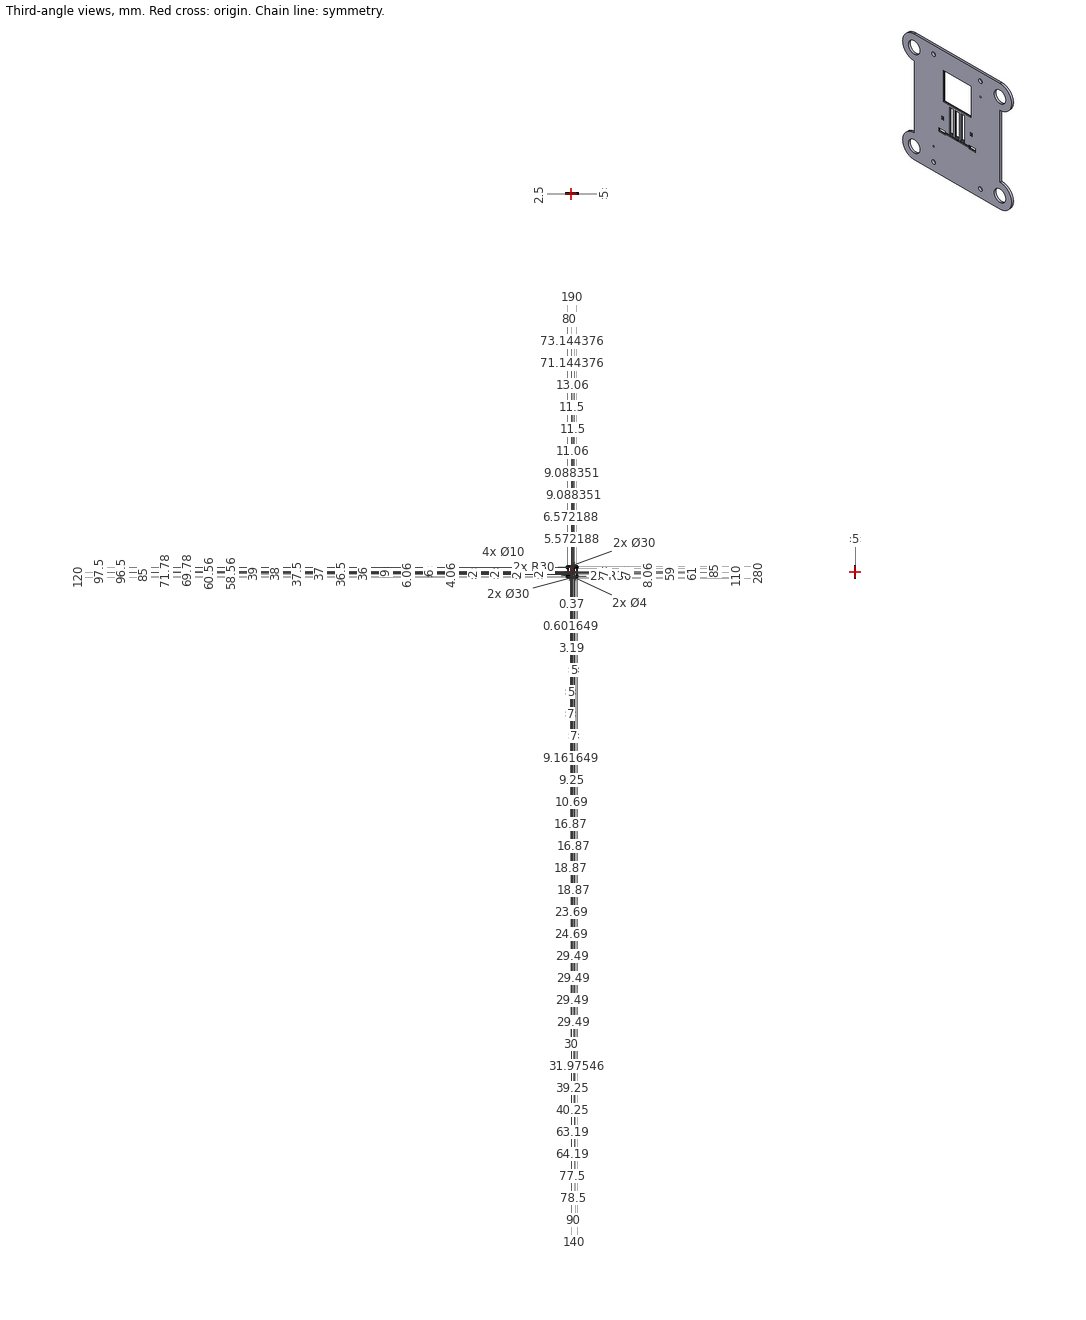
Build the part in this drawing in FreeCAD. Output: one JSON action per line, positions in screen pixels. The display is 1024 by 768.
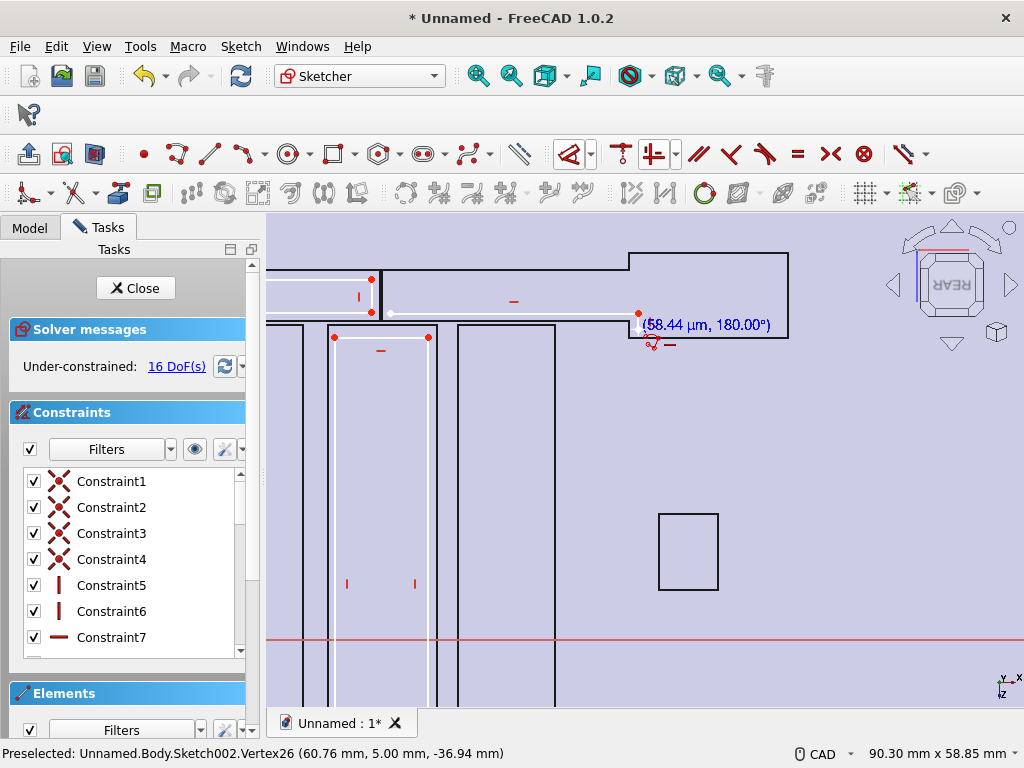
{"action": "scroll", "coordinate": [641, 330], "scroll_direction": "down", "scroll_amount": 7}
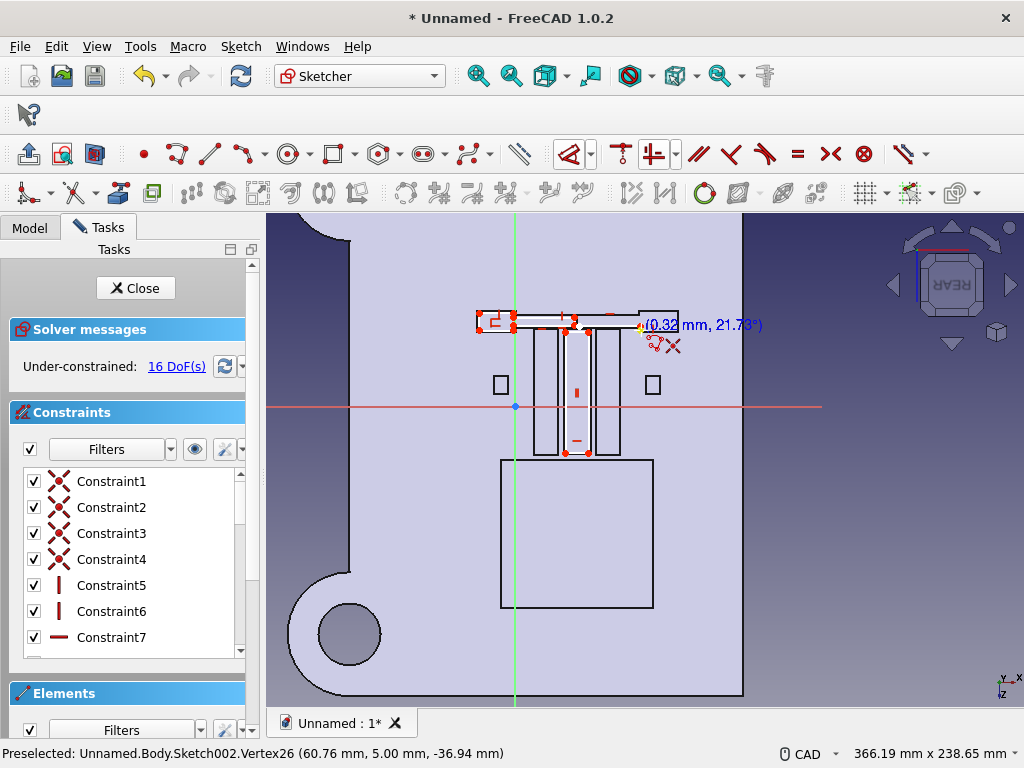
{"action": "left_click", "coordinate": [676, 330]}
{"action": "left_click", "coordinate": [676, 313]}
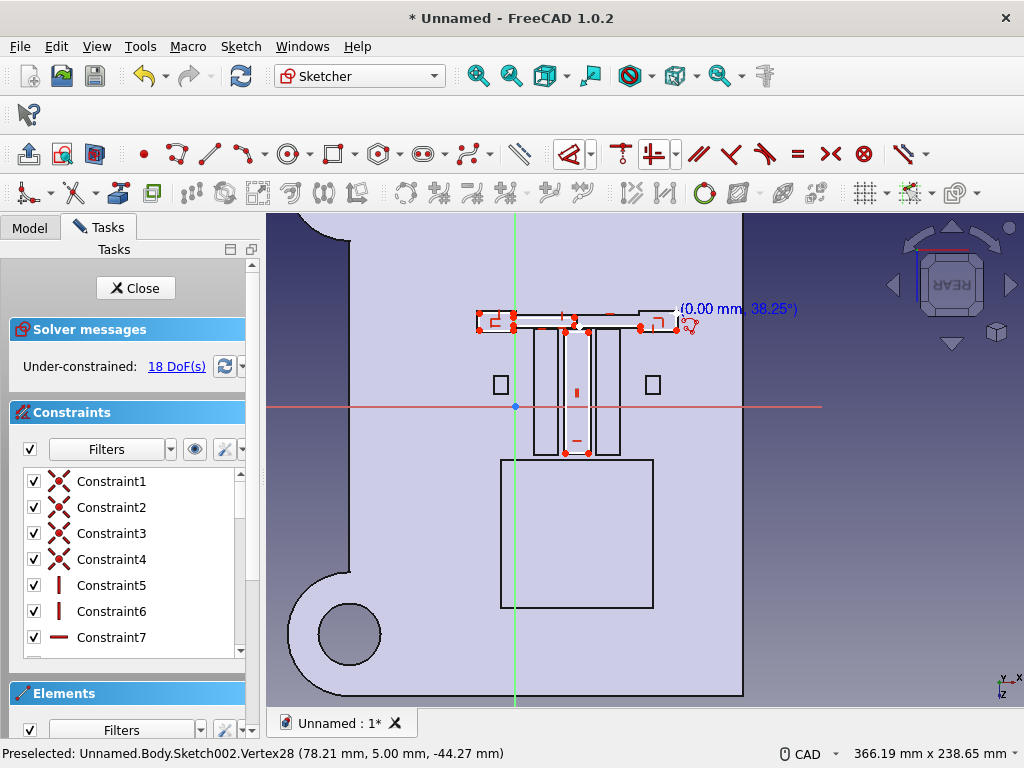
{"action": "scroll", "coordinate": [641, 313], "scroll_direction": "up", "scroll_amount": 2}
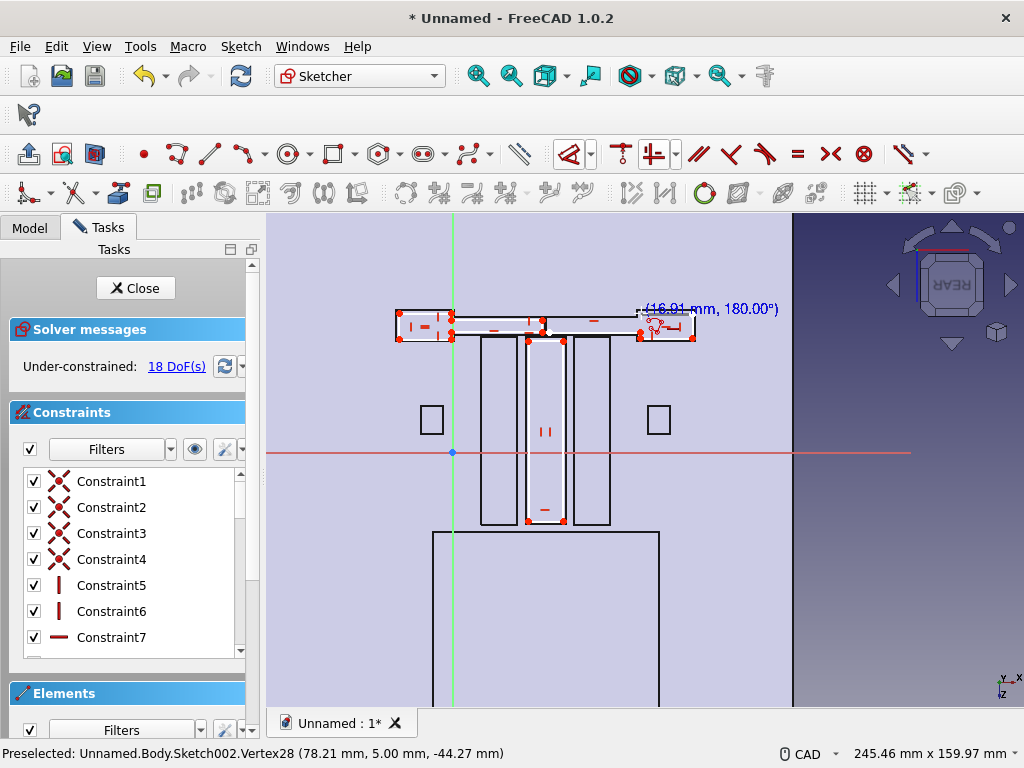
{"action": "left_click", "coordinate": [640, 313]}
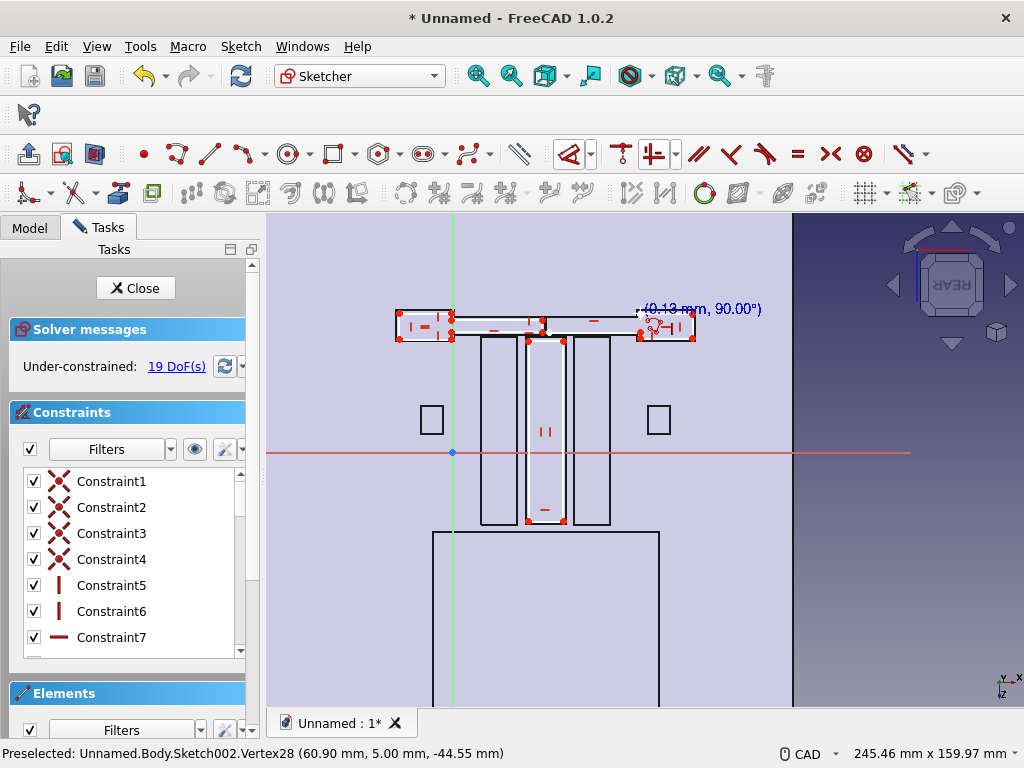
{"action": "scroll", "coordinate": [640, 320], "scroll_direction": "up", "scroll_amount": 5}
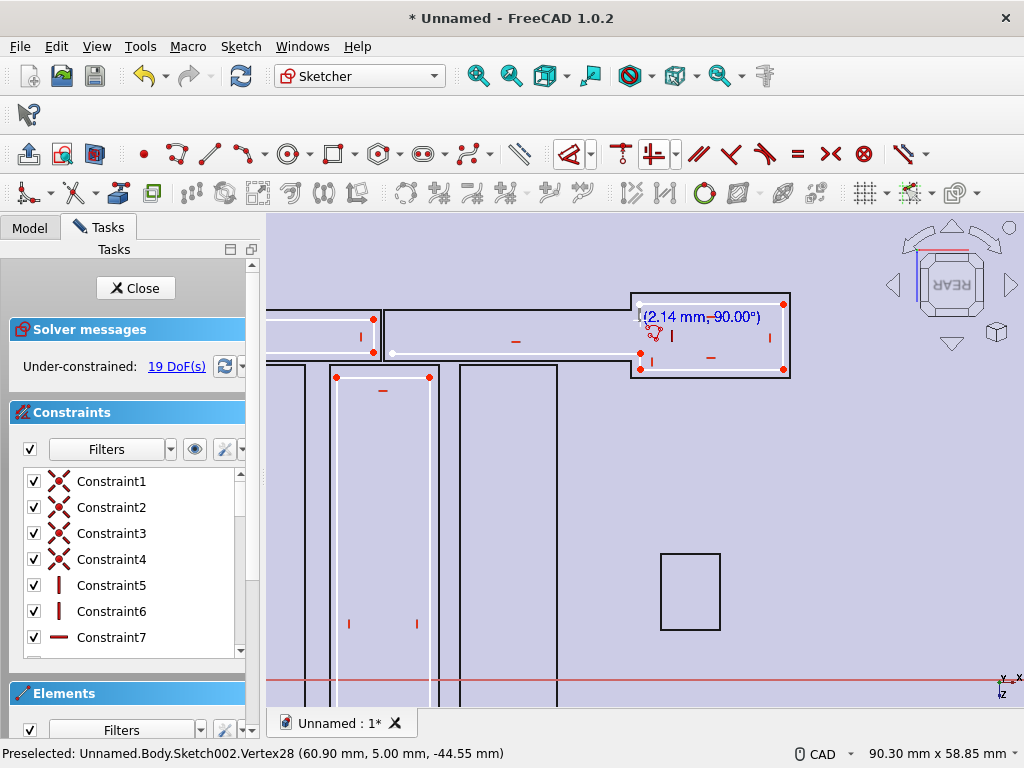
{"action": "left_click", "coordinate": [639, 319]}
{"action": "left_click", "coordinate": [392, 319]}
{"action": "left_click", "coordinate": [392, 354]}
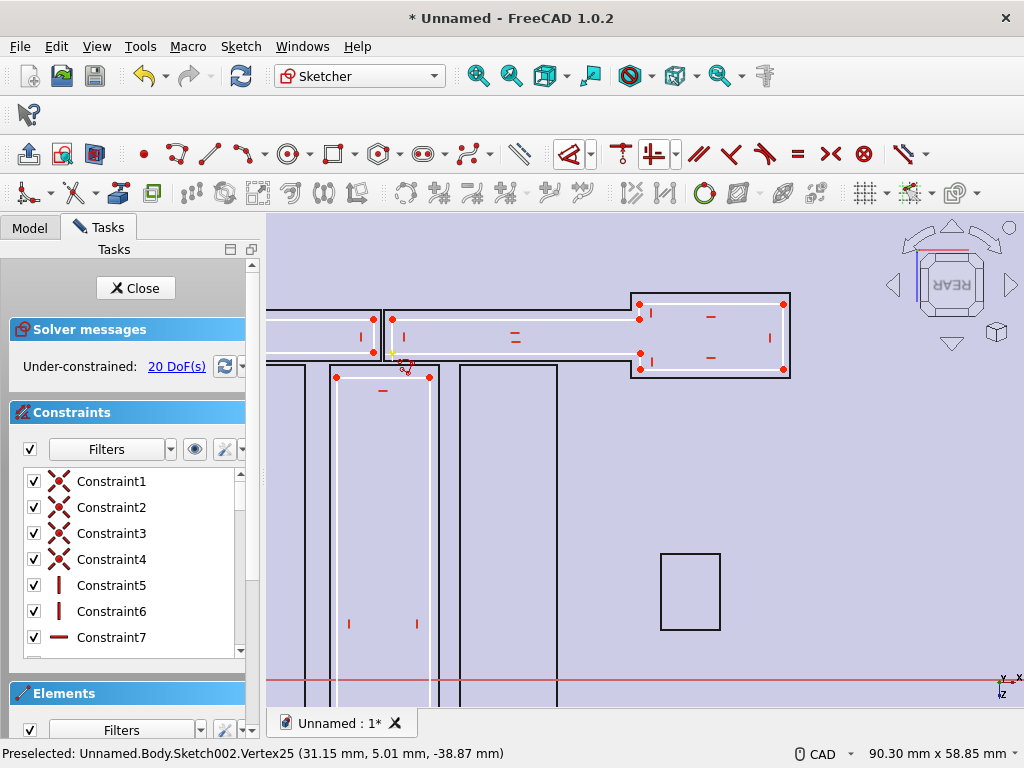
{"action": "left_click", "coordinate": [332, 154]}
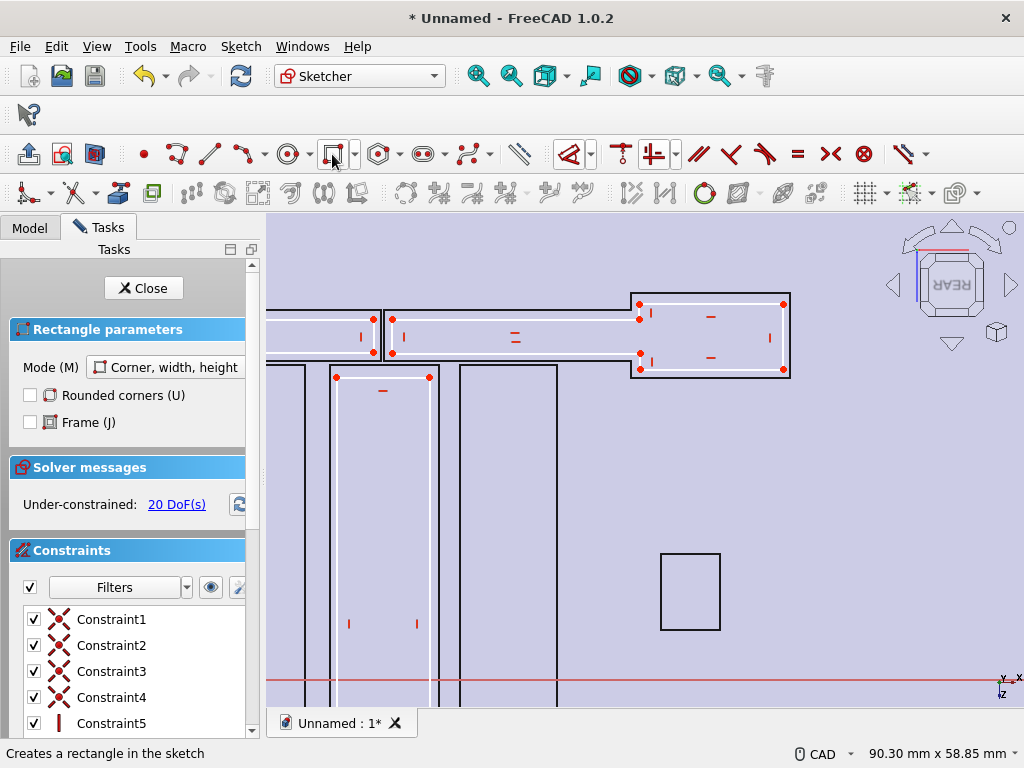
{"action": "left_click", "coordinate": [469, 374]}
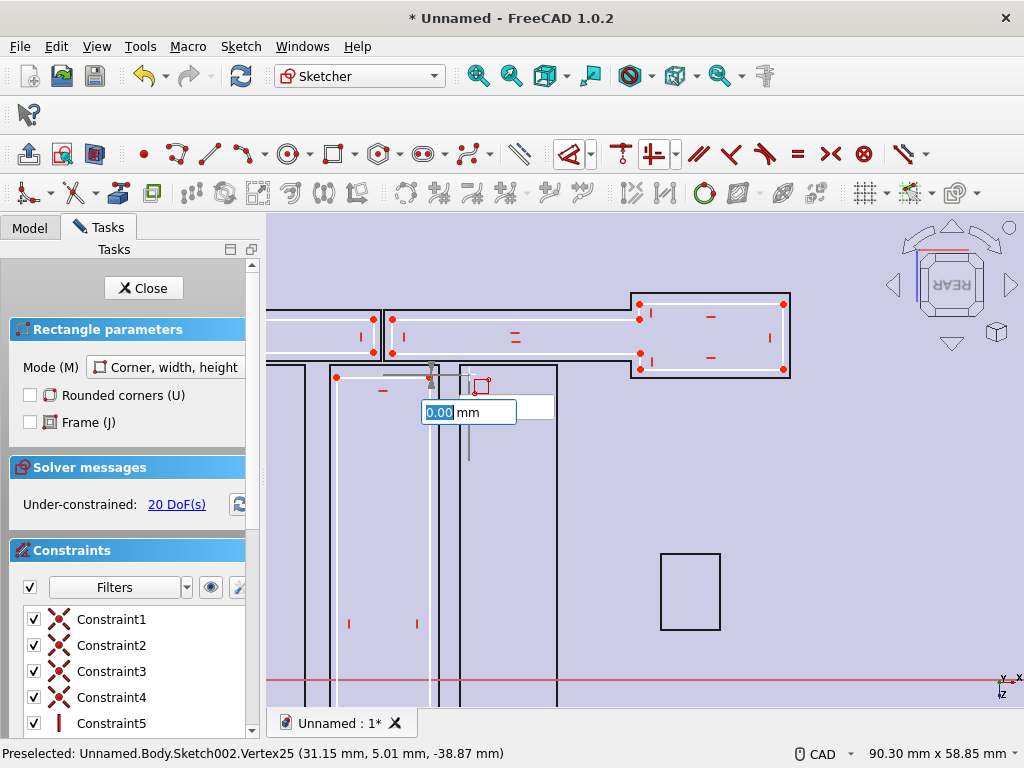
{"action": "scroll", "coordinate": [640, 317], "scroll_direction": "down", "scroll_amount": 7}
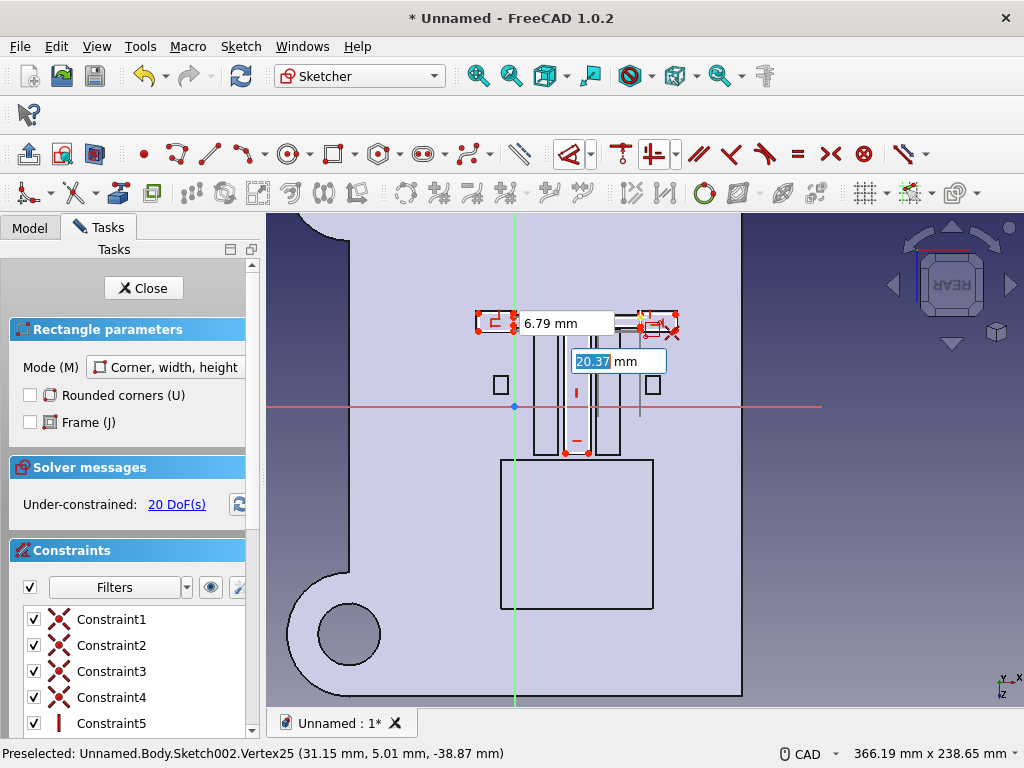
{"action": "left_click", "coordinate": [617, 453]}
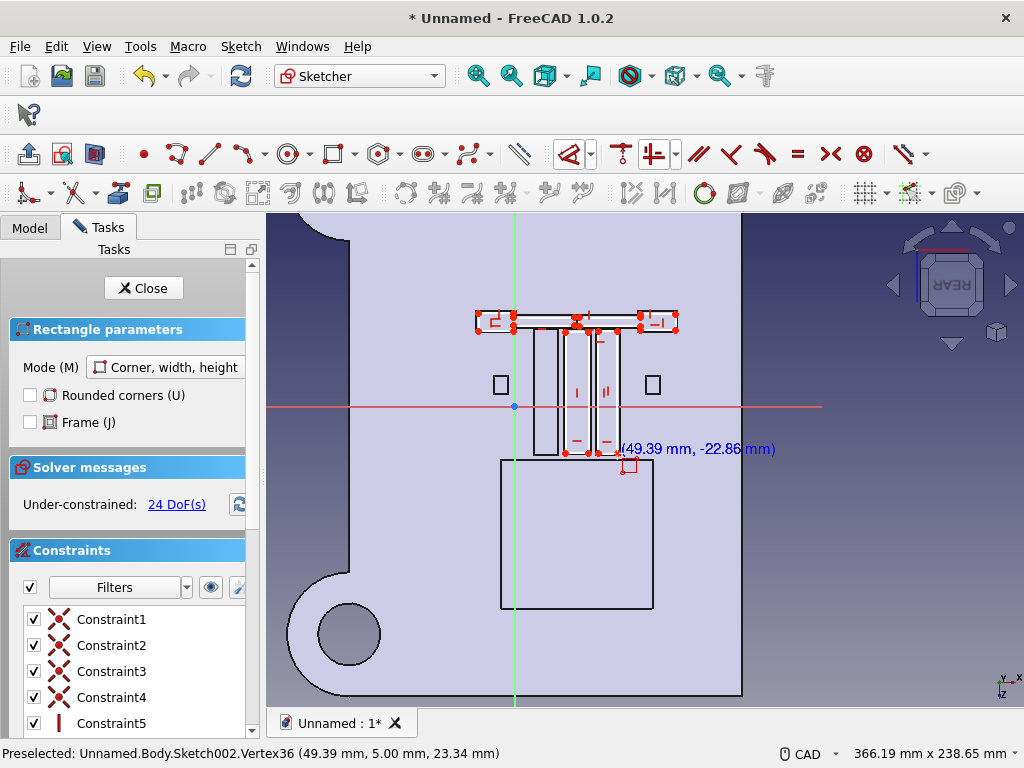
{"action": "scroll", "coordinate": [648, 378], "scroll_direction": "up", "scroll_amount": 3}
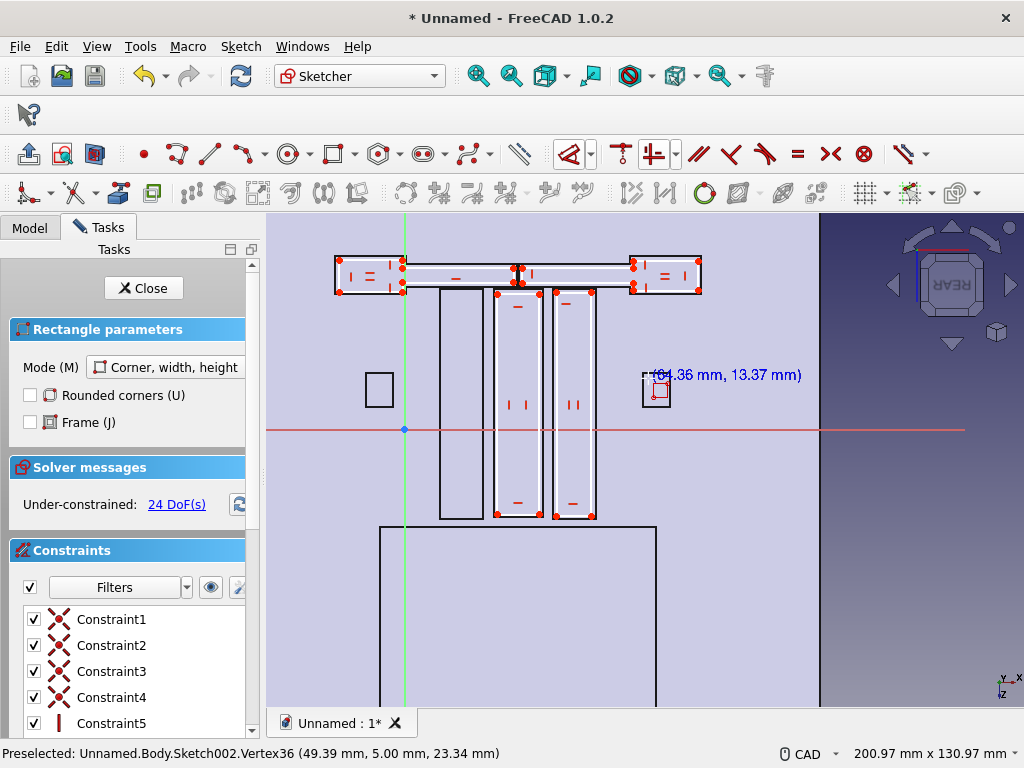
{"action": "left_click", "coordinate": [647, 377]}
{"action": "left_click", "coordinate": [666, 404]}